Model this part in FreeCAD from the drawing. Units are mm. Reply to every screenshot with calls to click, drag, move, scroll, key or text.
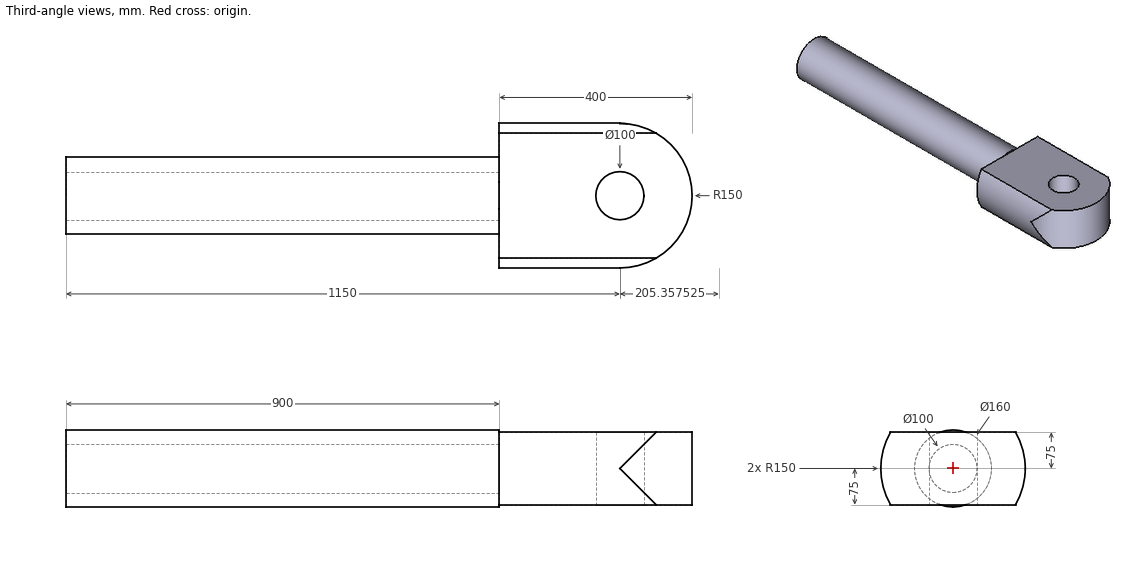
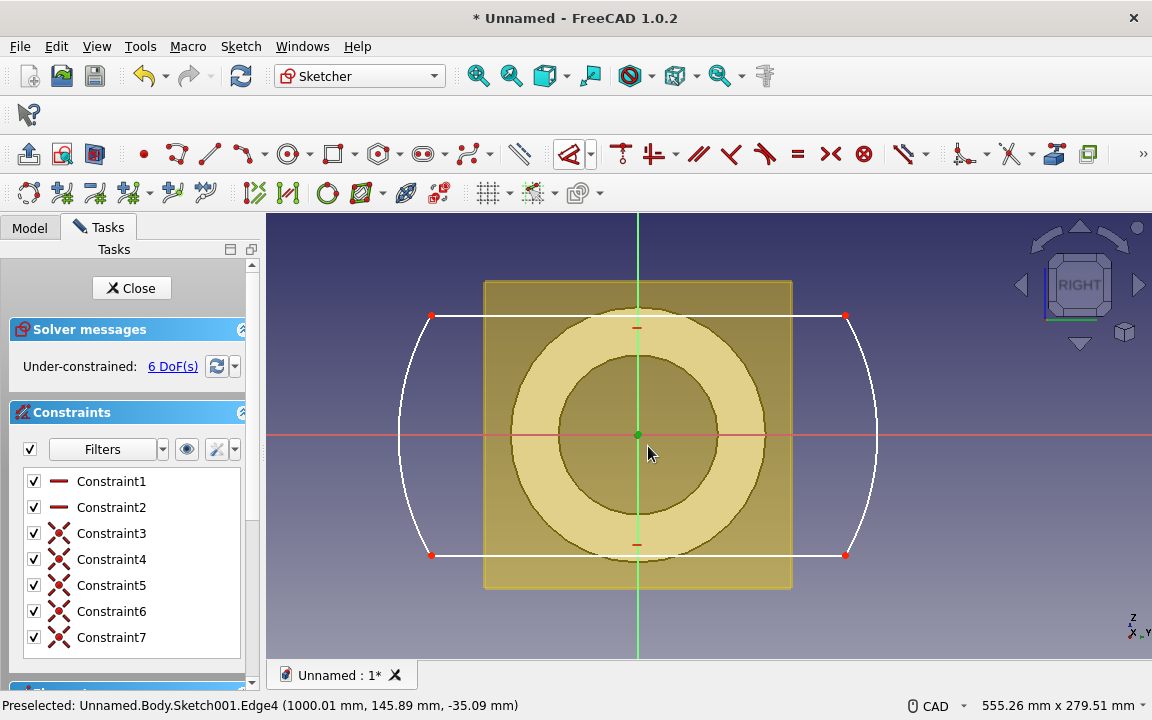
key(c)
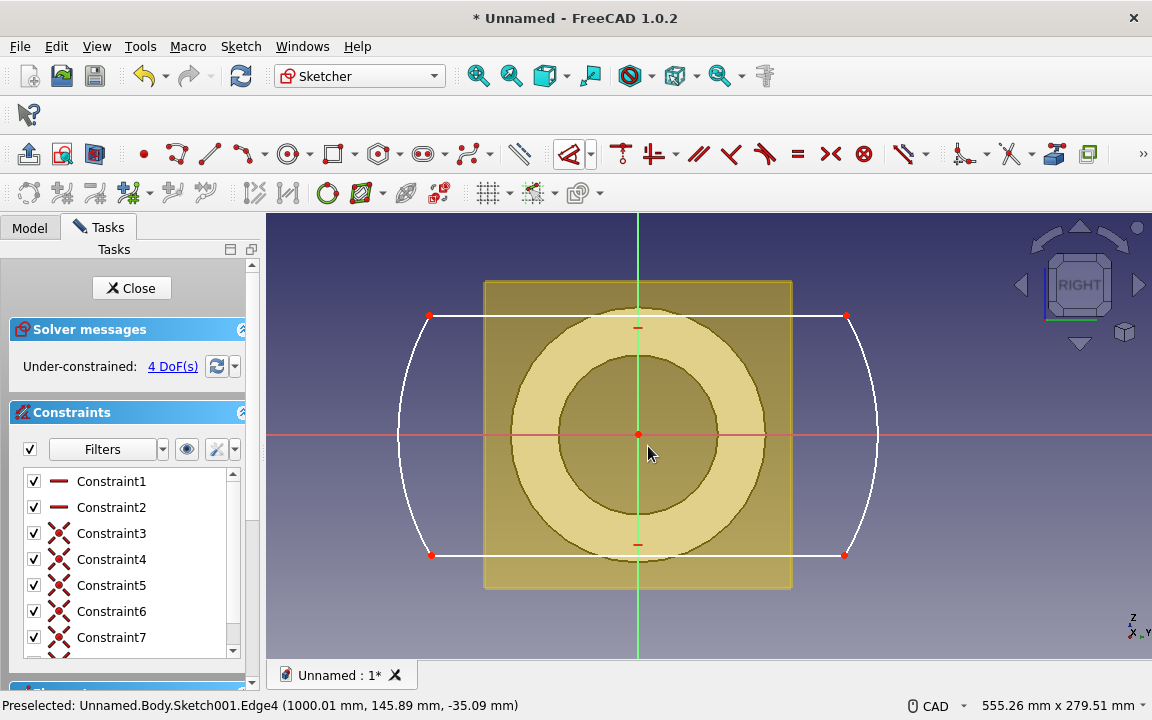
click(403, 386)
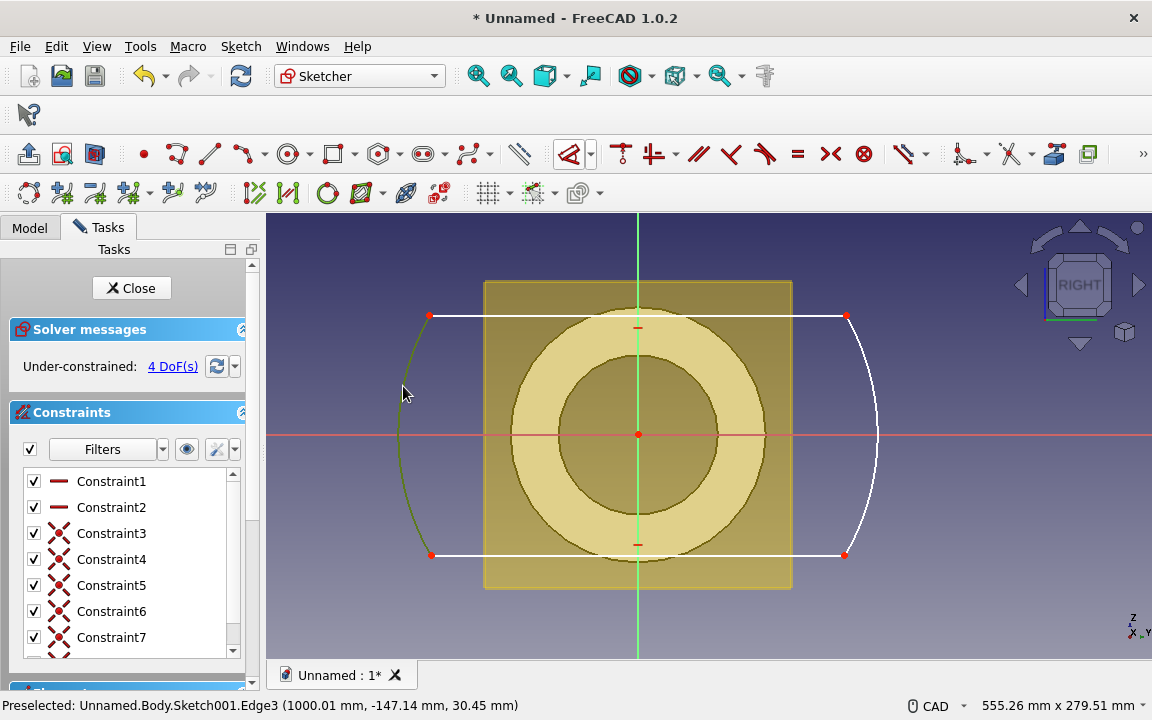
click(872, 486)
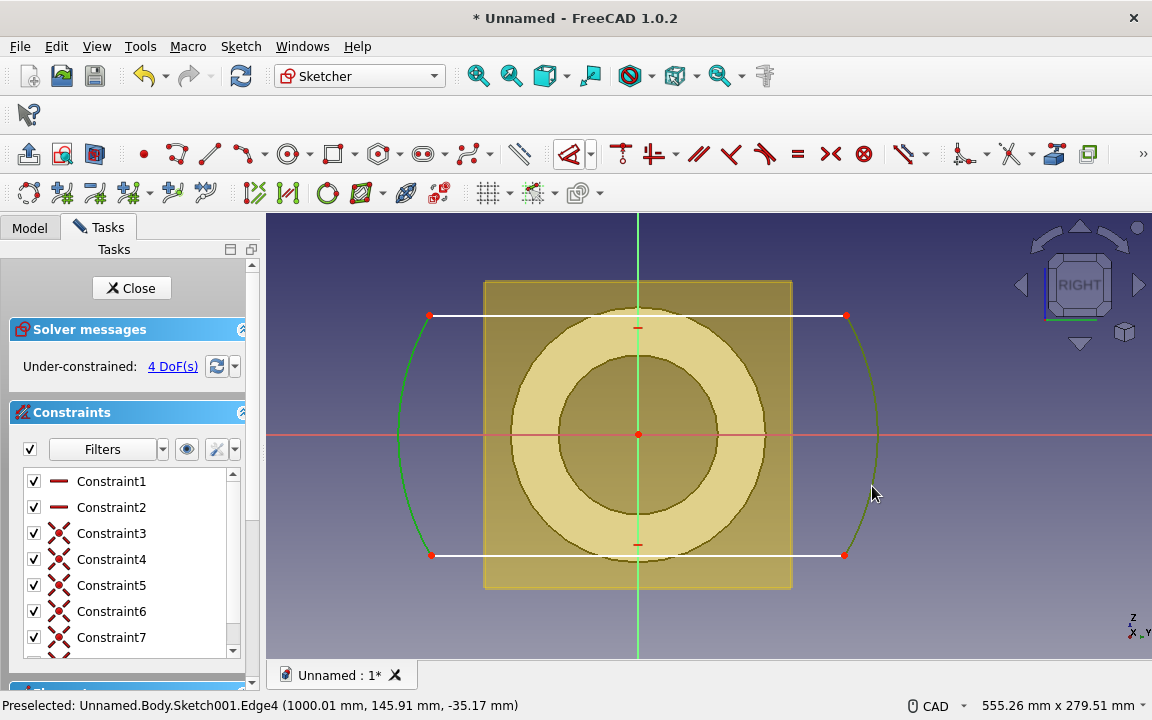
key(e)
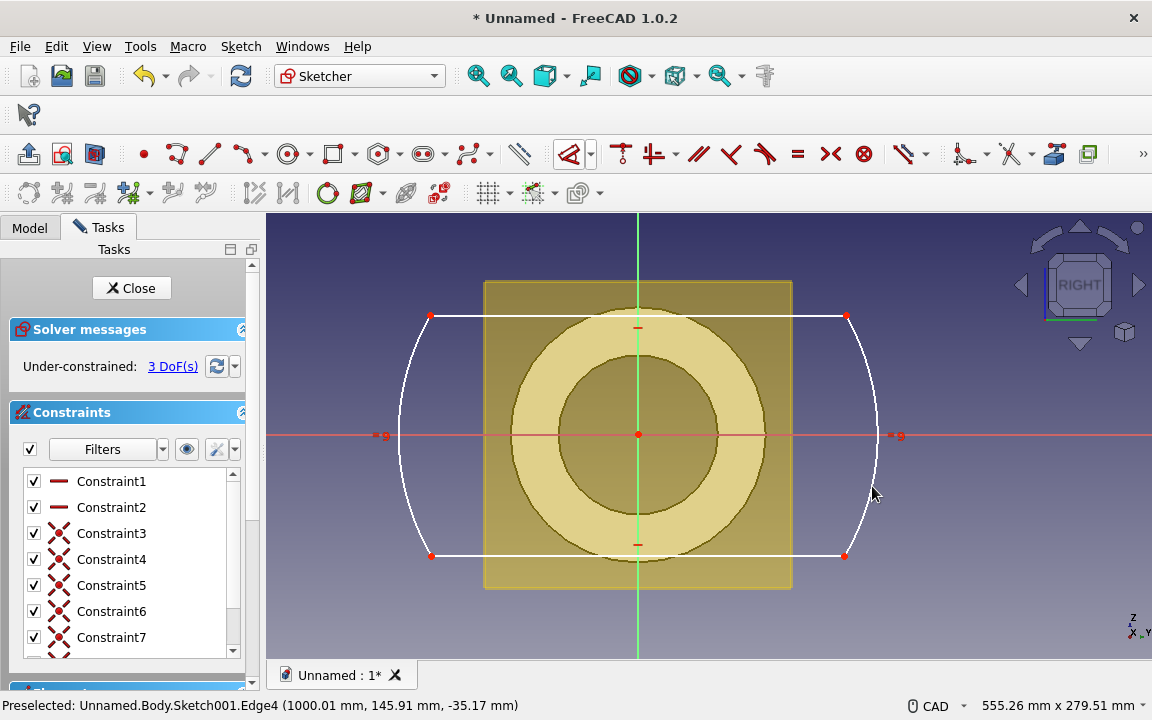
key(d)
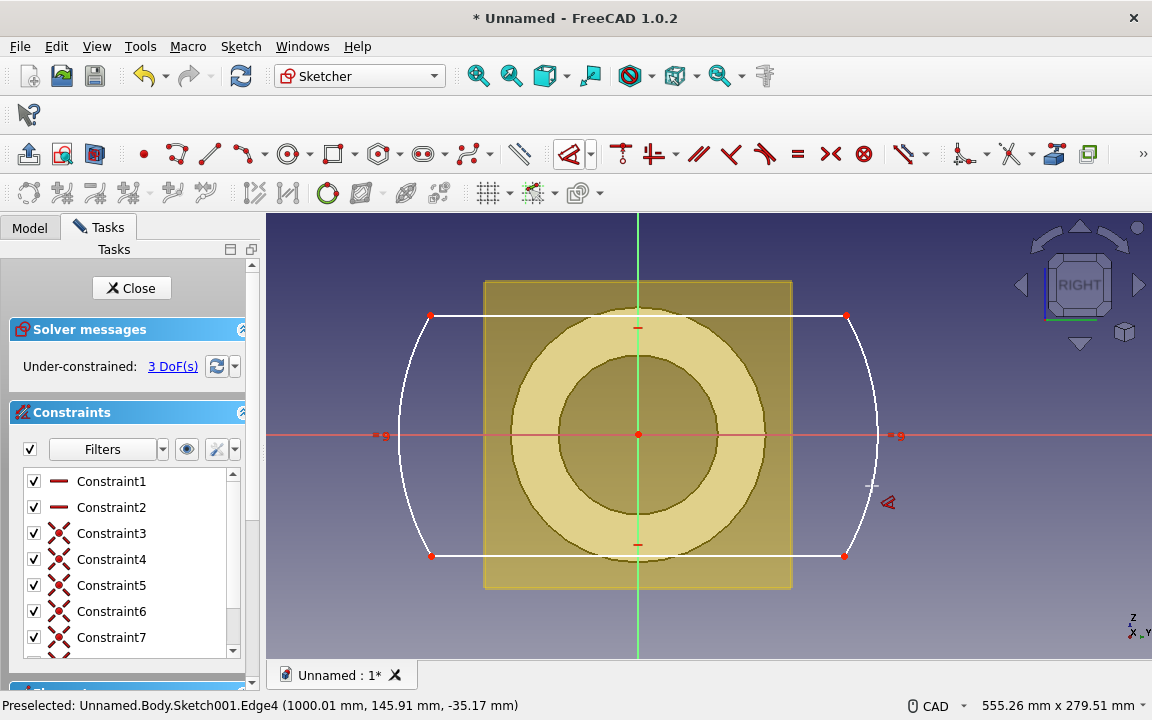
click(404, 386)
click(373, 379)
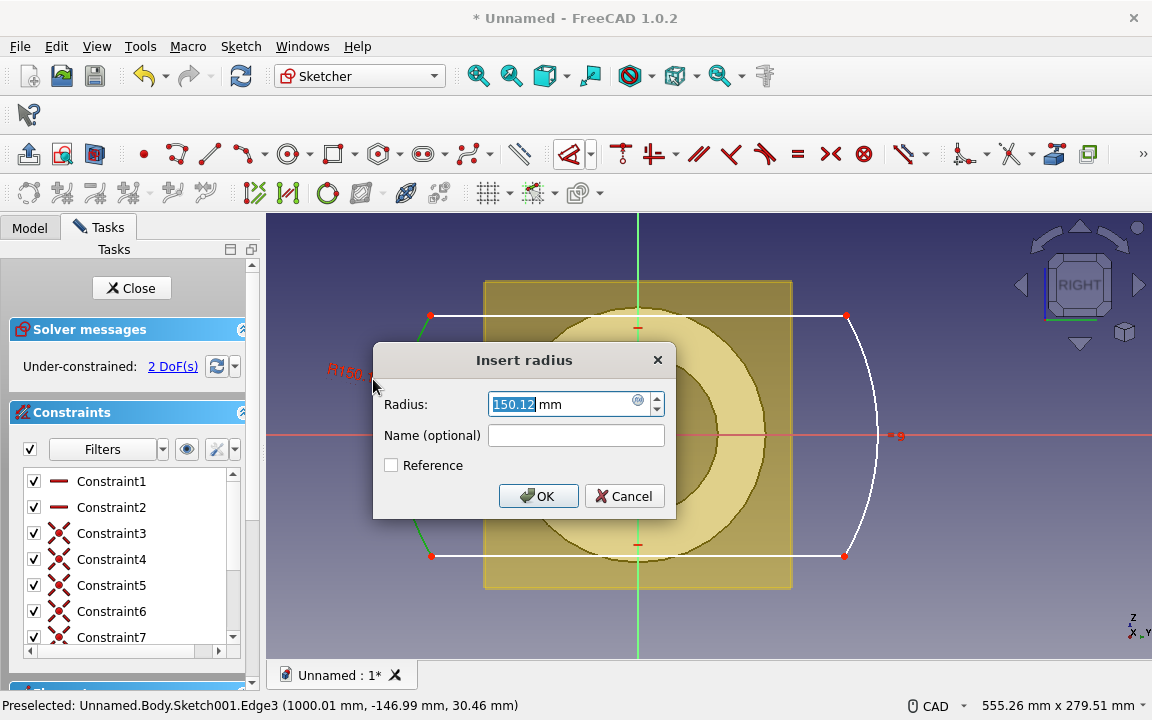
text(150)
key(Return)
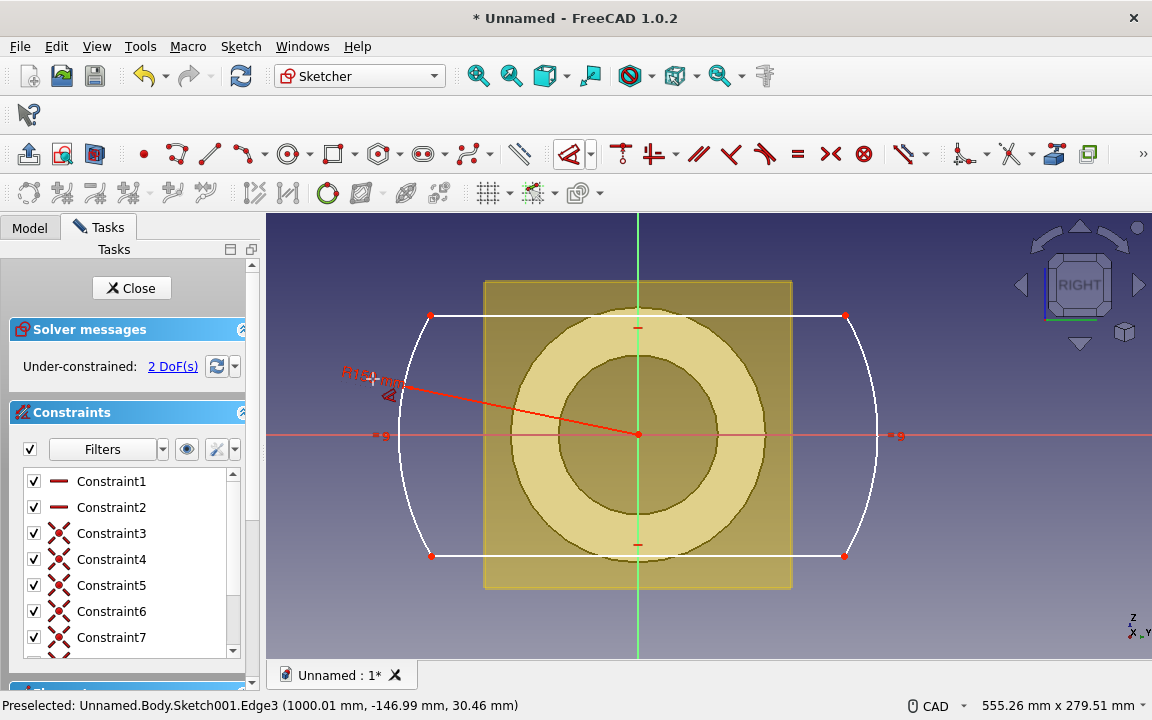
click(846, 316)
click(880, 348)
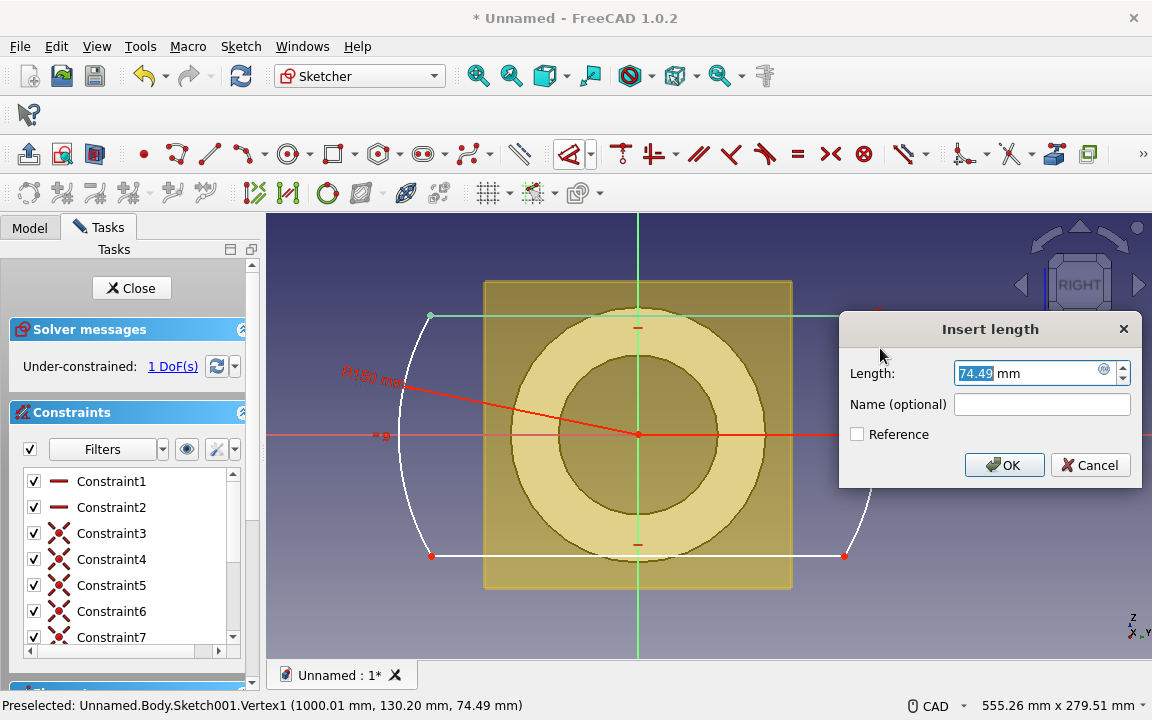
text(75)
key(Return)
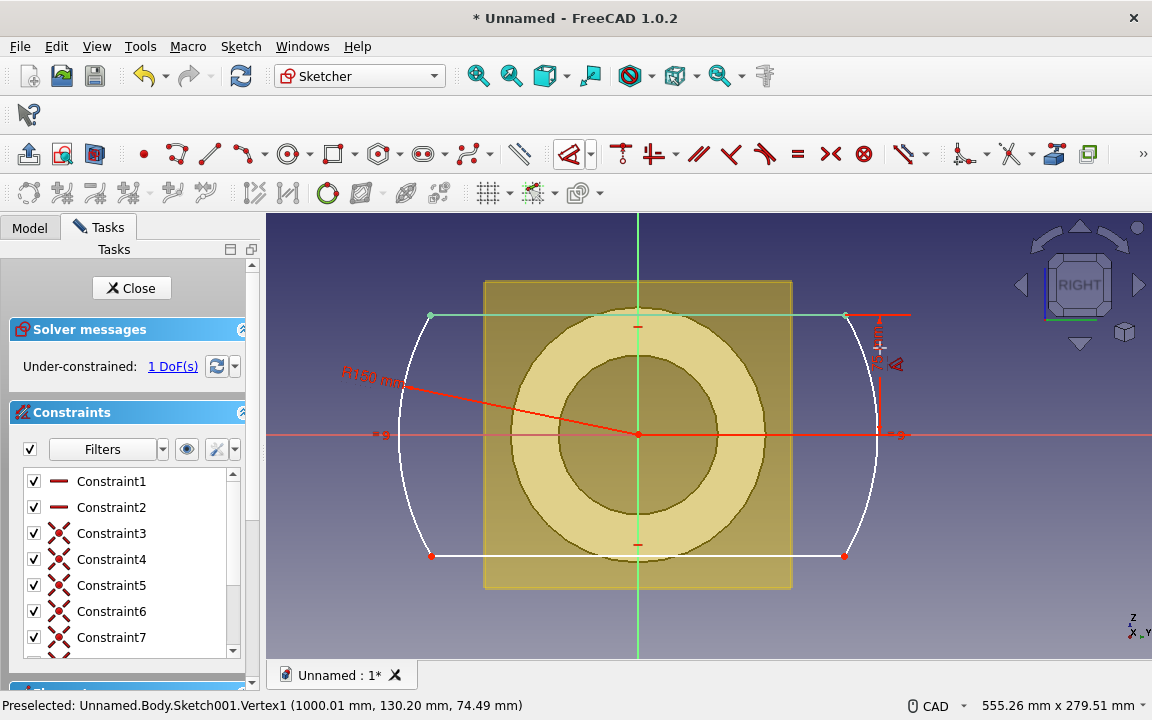
click(432, 556)
click(398, 523)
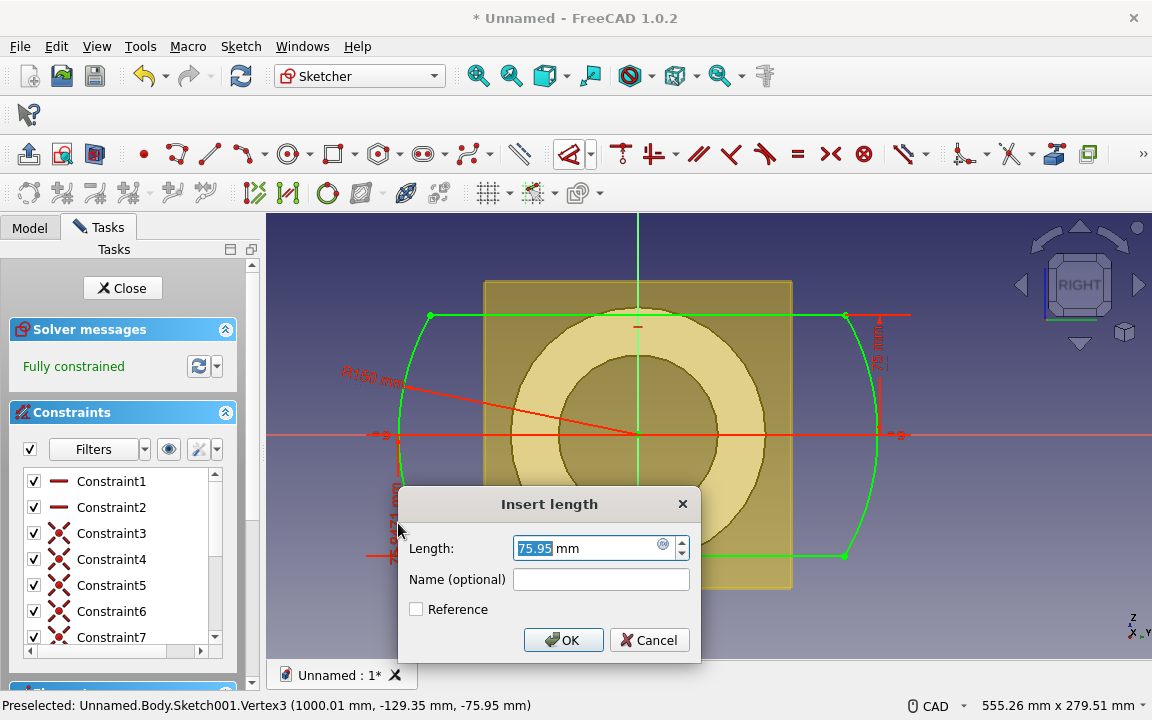
text(75)
key(Return)
key(Escape)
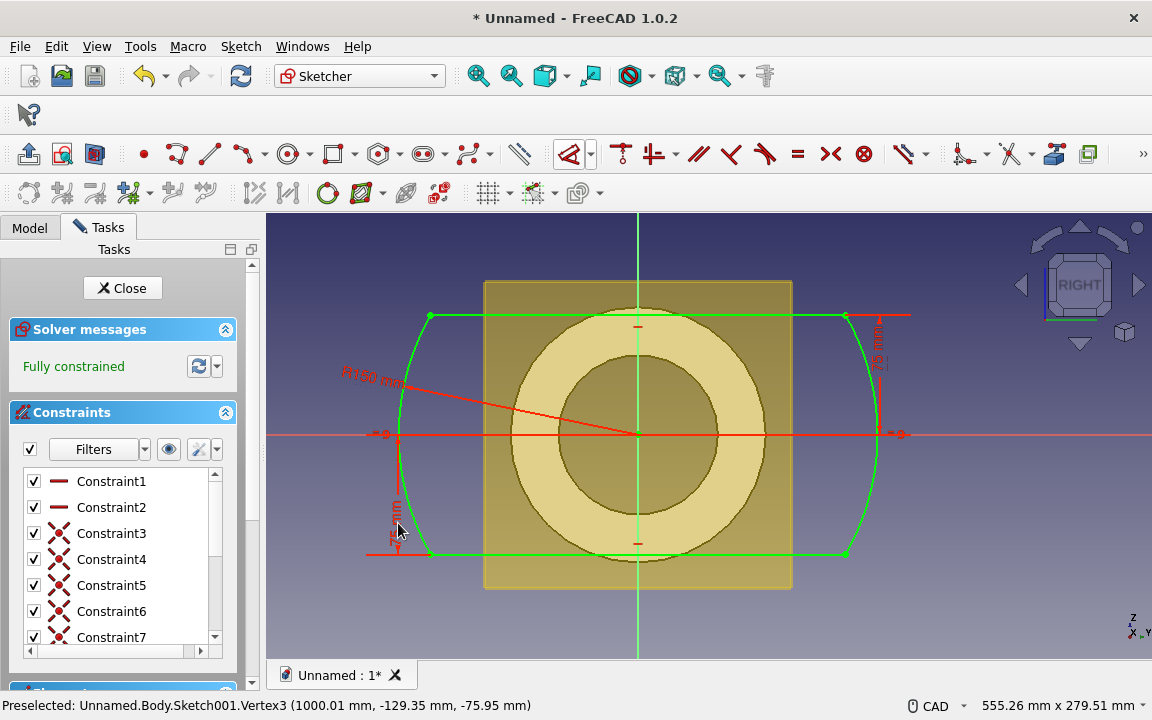
click(123, 288)